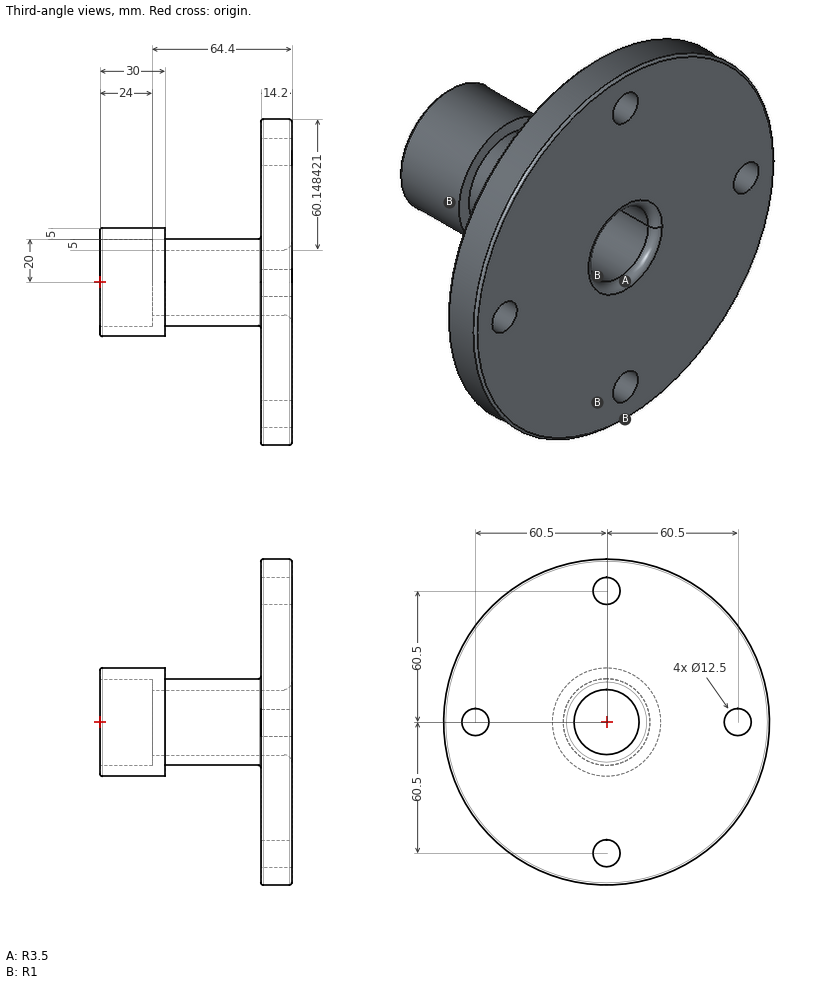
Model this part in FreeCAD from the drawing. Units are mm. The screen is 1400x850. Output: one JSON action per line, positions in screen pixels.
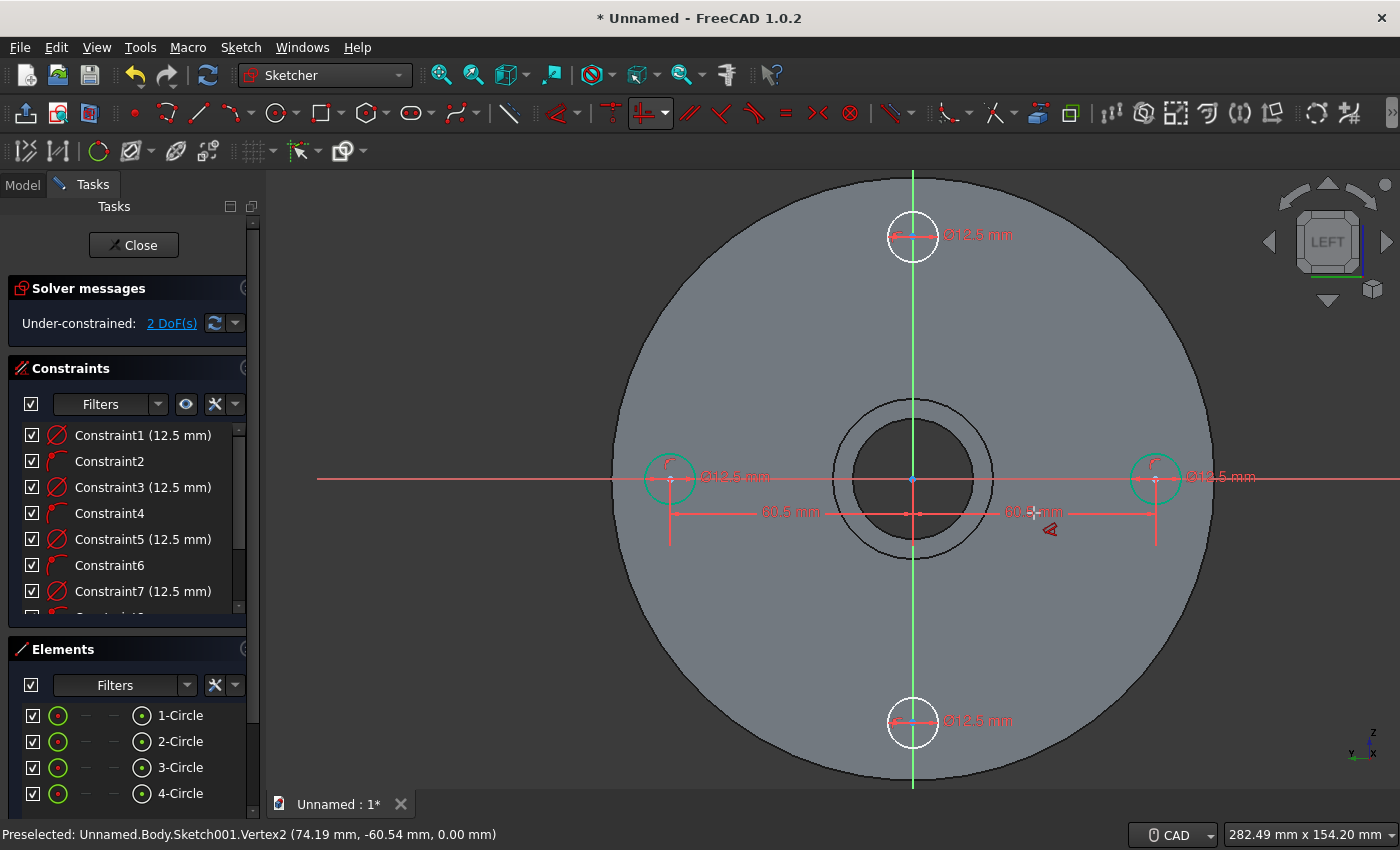
{"action": "left_click", "coordinate": [913, 723]}
{"action": "left_click", "coordinate": [947, 601]}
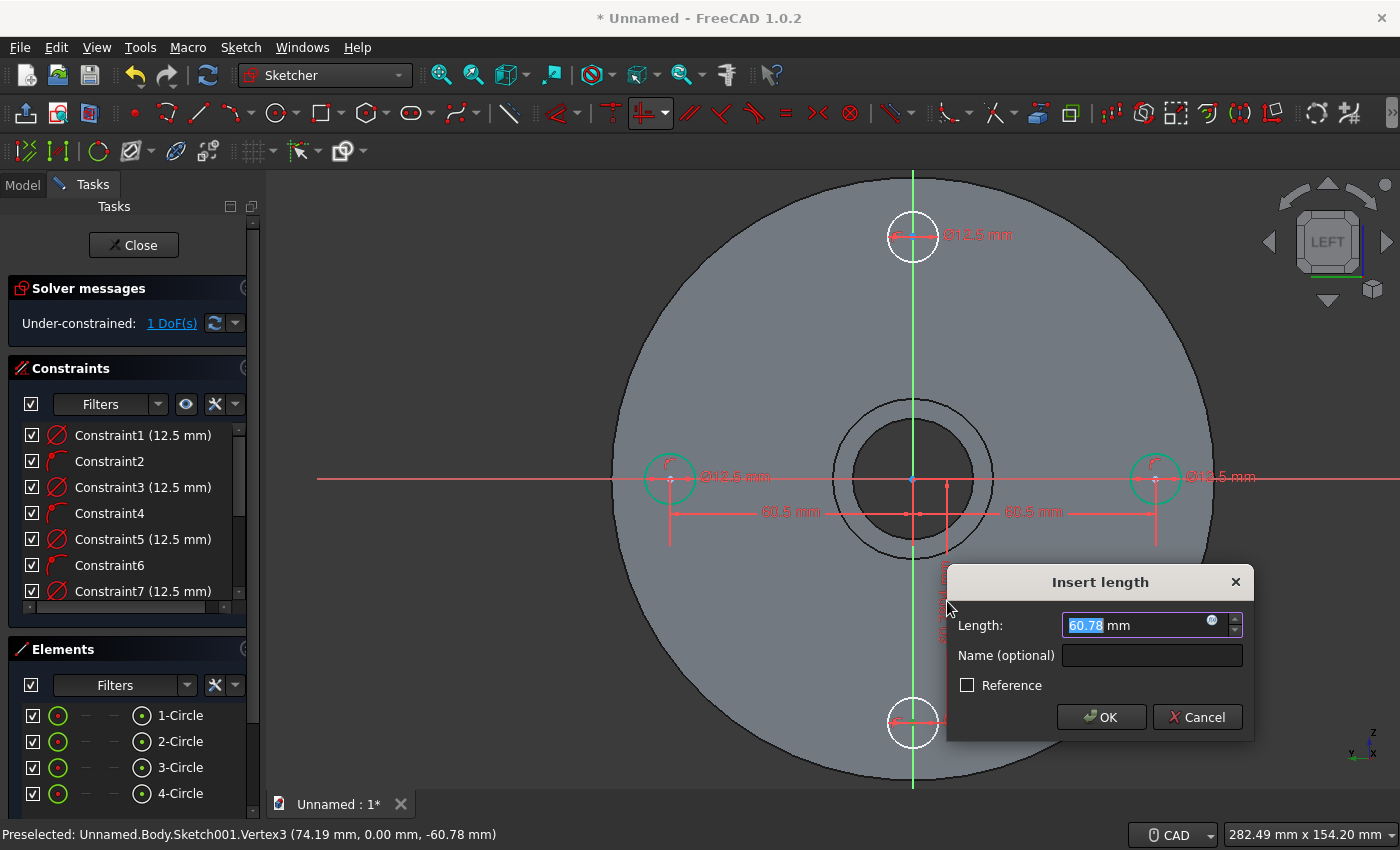
{"action": "type", "text": "60.5"}
{"action": "key", "text": "Return"}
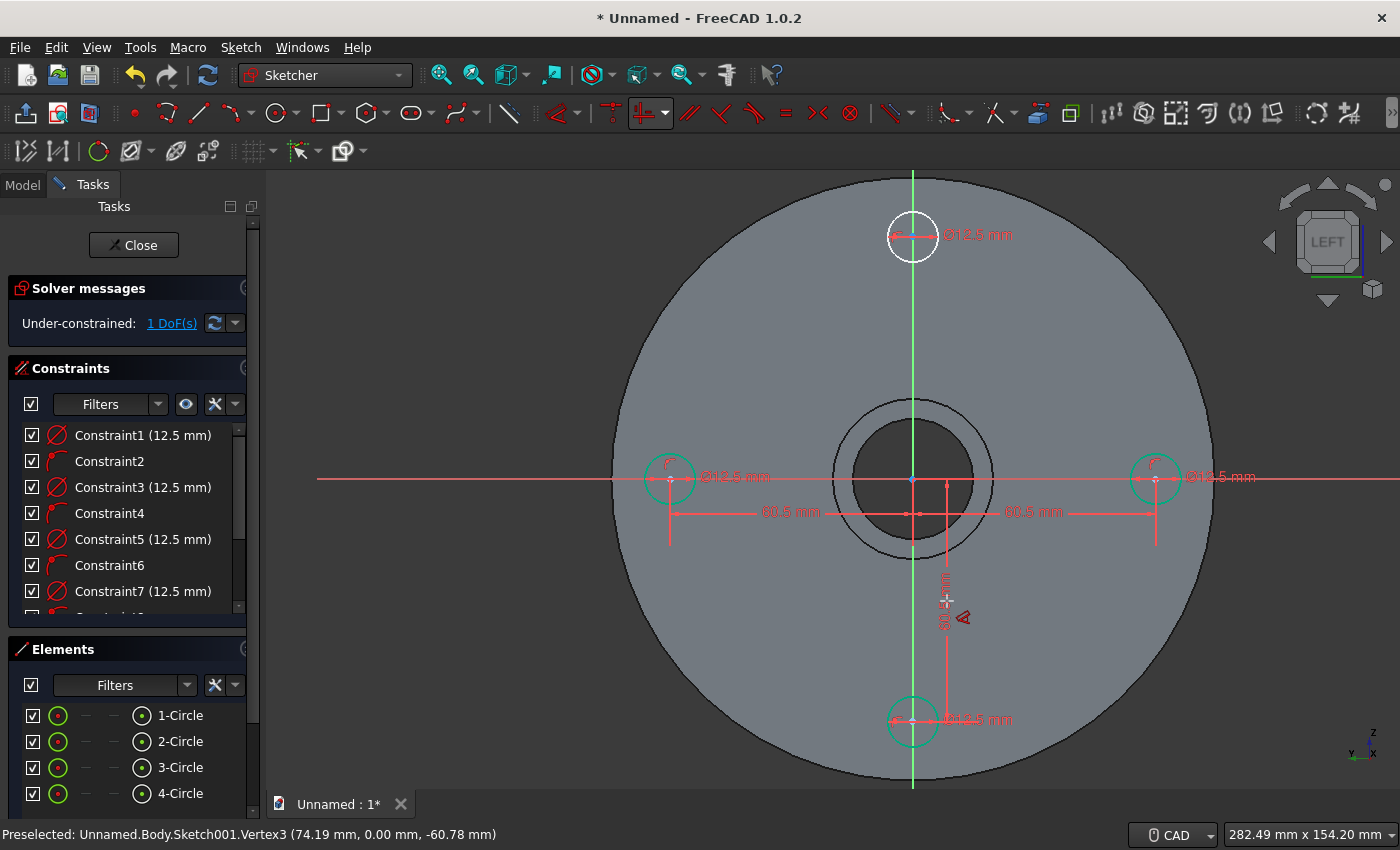
{"action": "left_click", "coordinate": [913, 237]}
{"action": "left_click", "coordinate": [947, 358]}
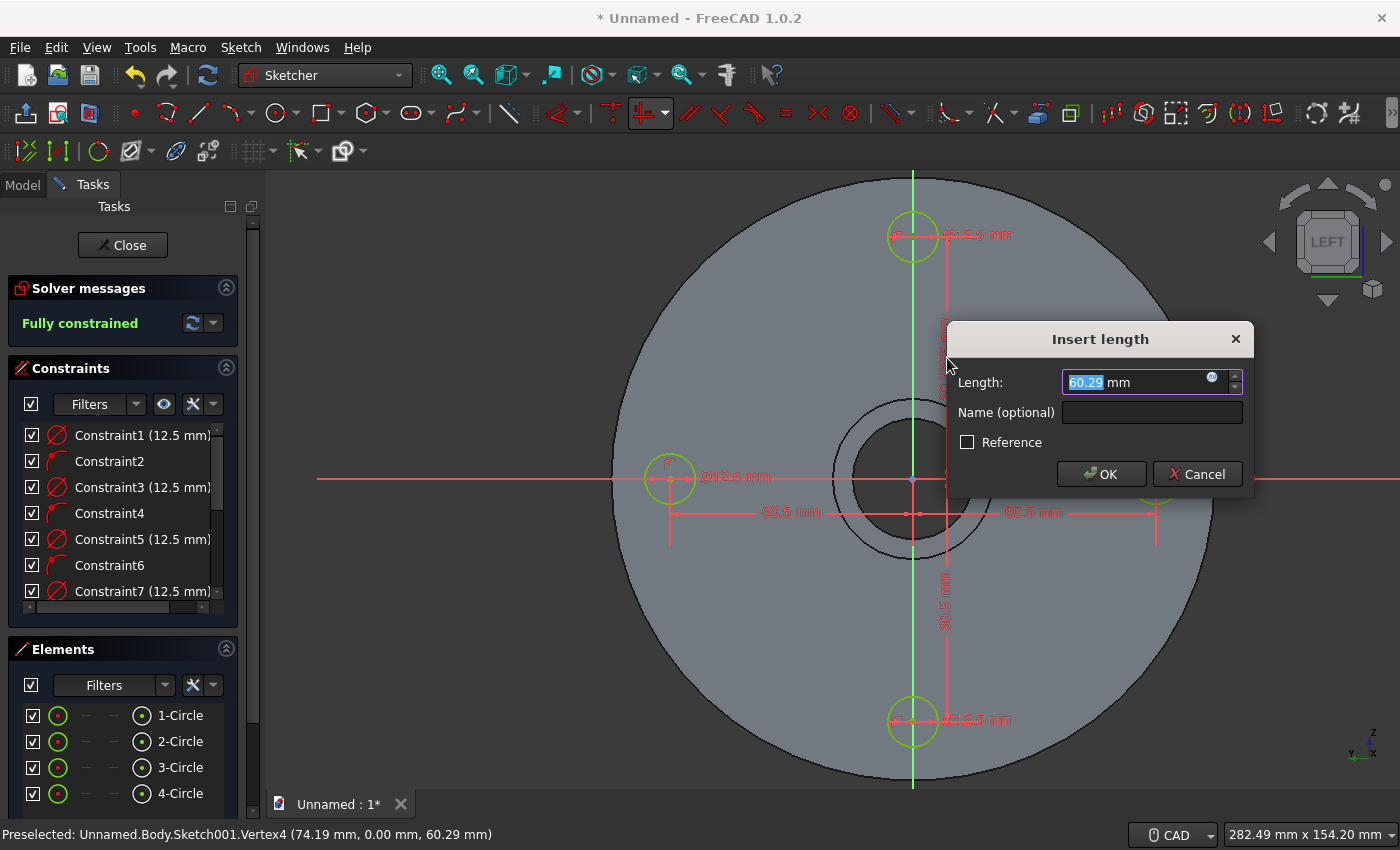
{"action": "type", "text": "60.5"}
{"action": "key", "text": "Return"}
{"action": "key", "text": "Escape"}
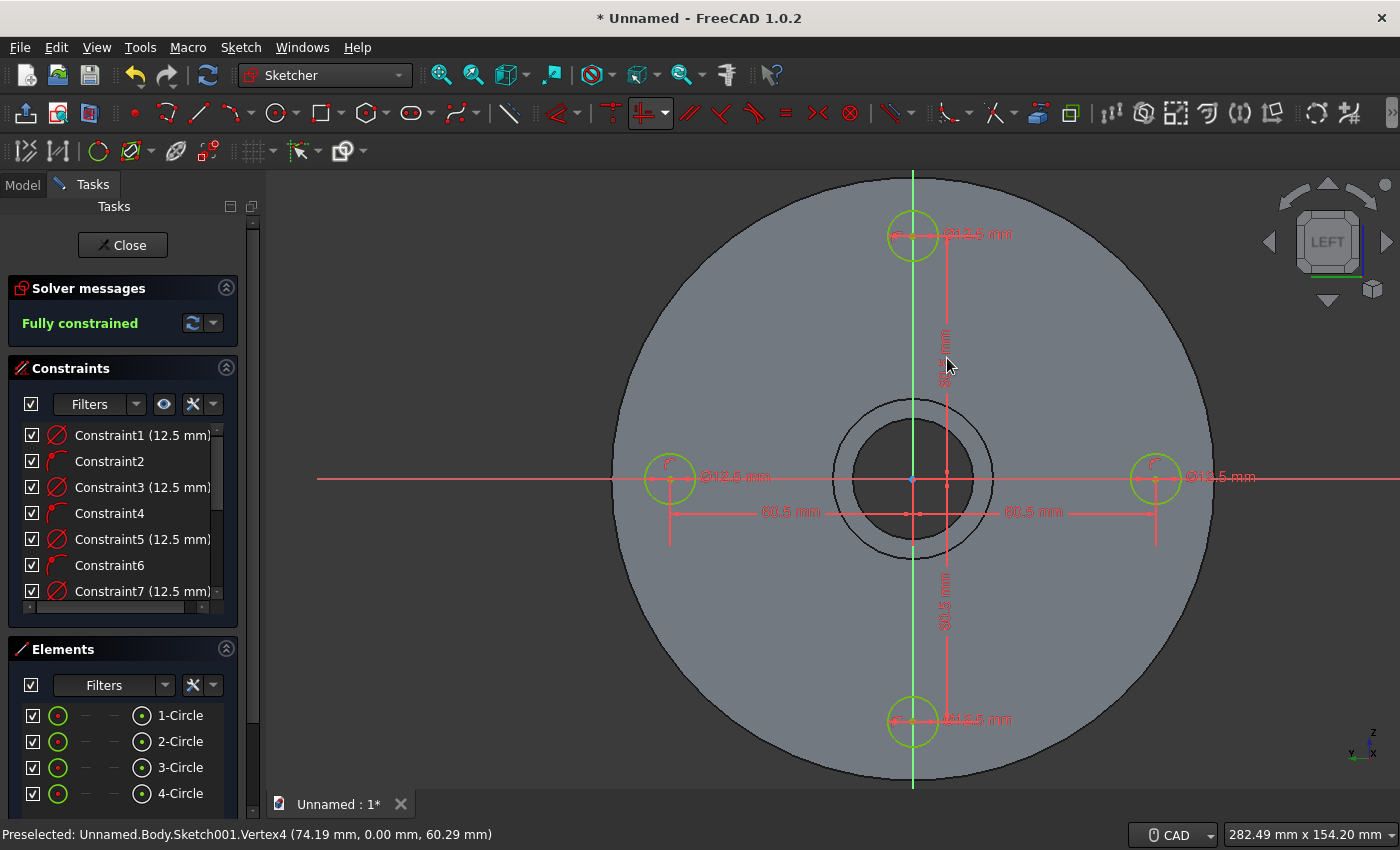
{"action": "left_click", "coordinate": [123, 245]}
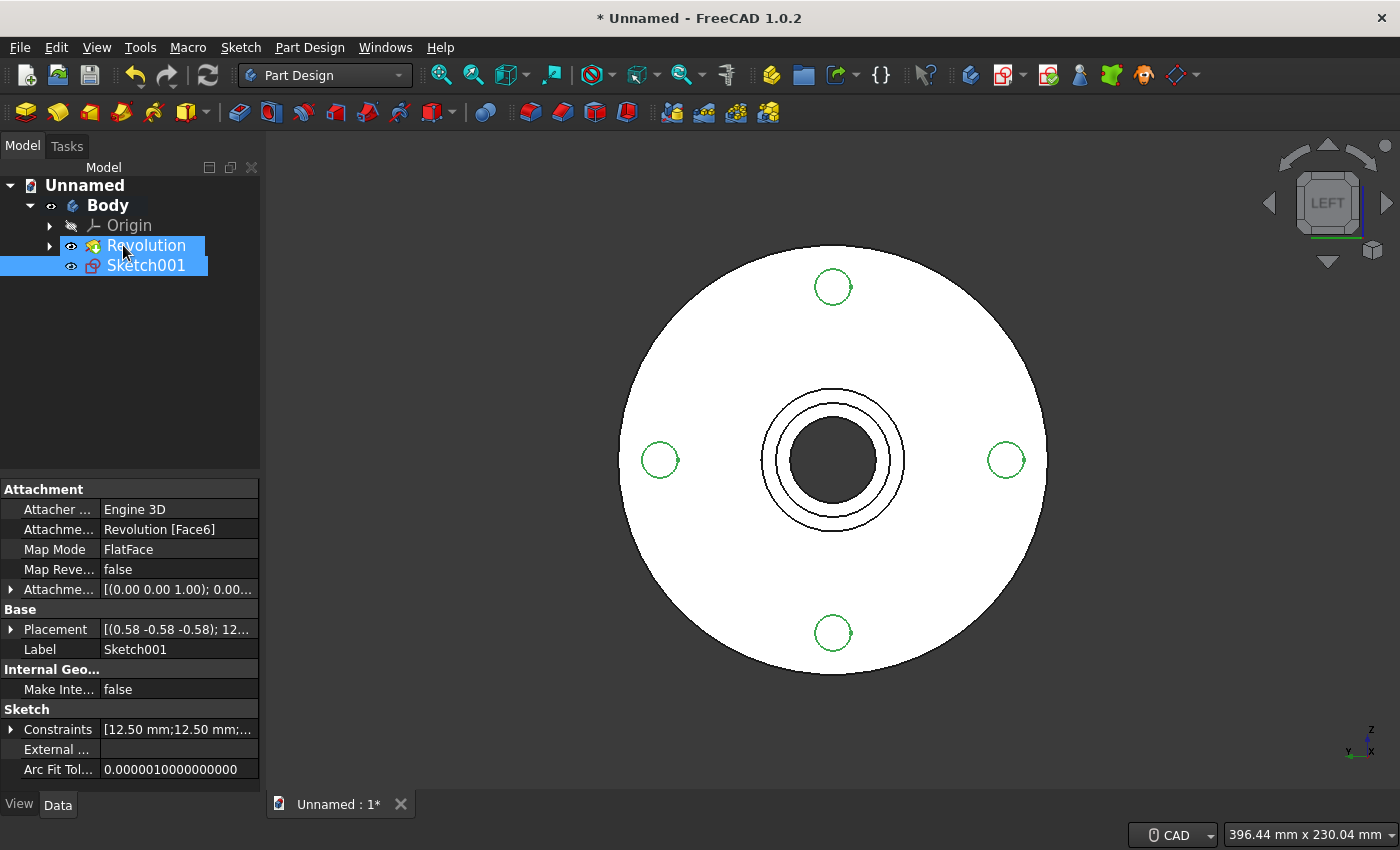
{"action": "left_click", "coordinate": [240, 112]}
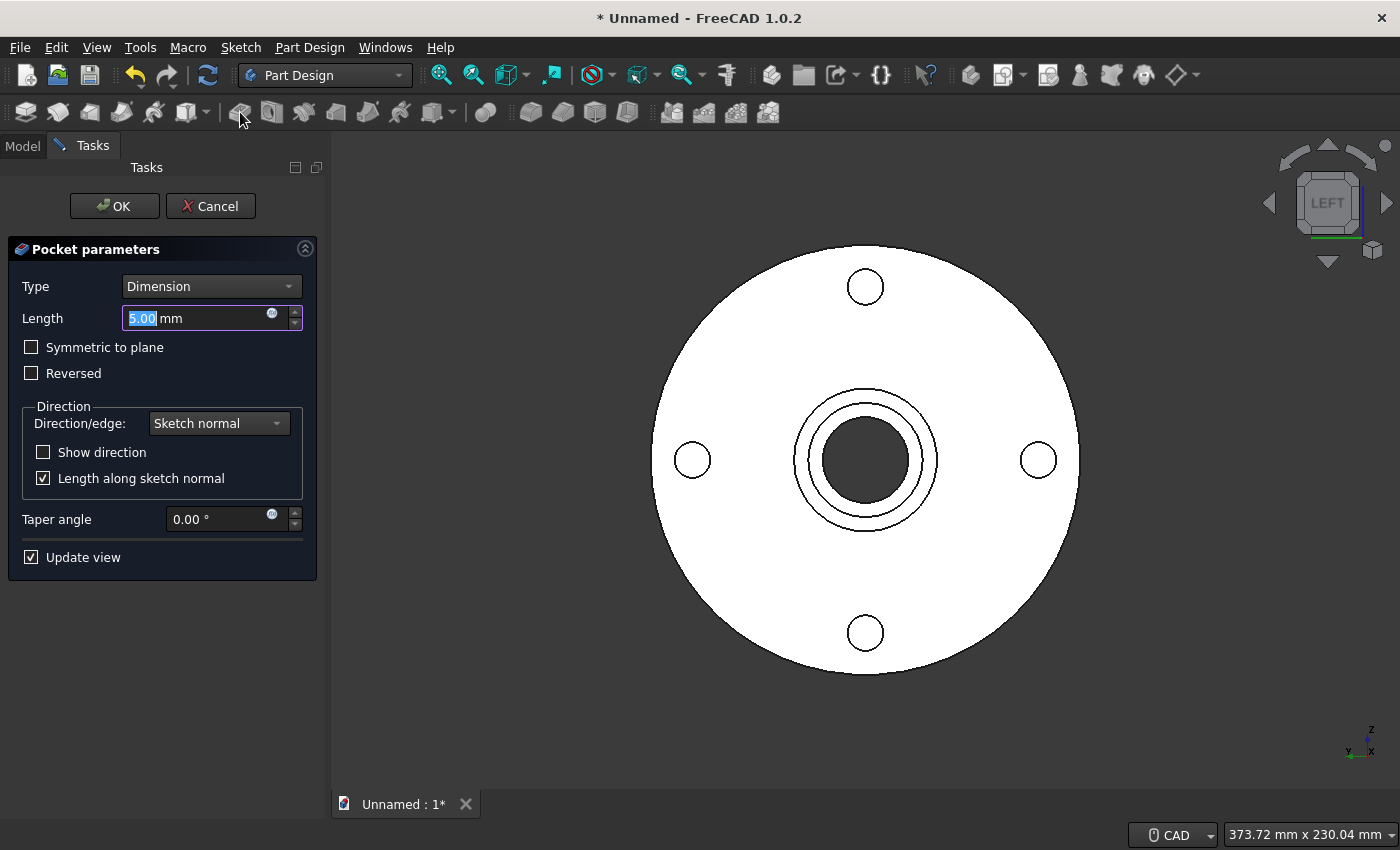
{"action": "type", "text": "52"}
{"action": "key", "text": "Tab"}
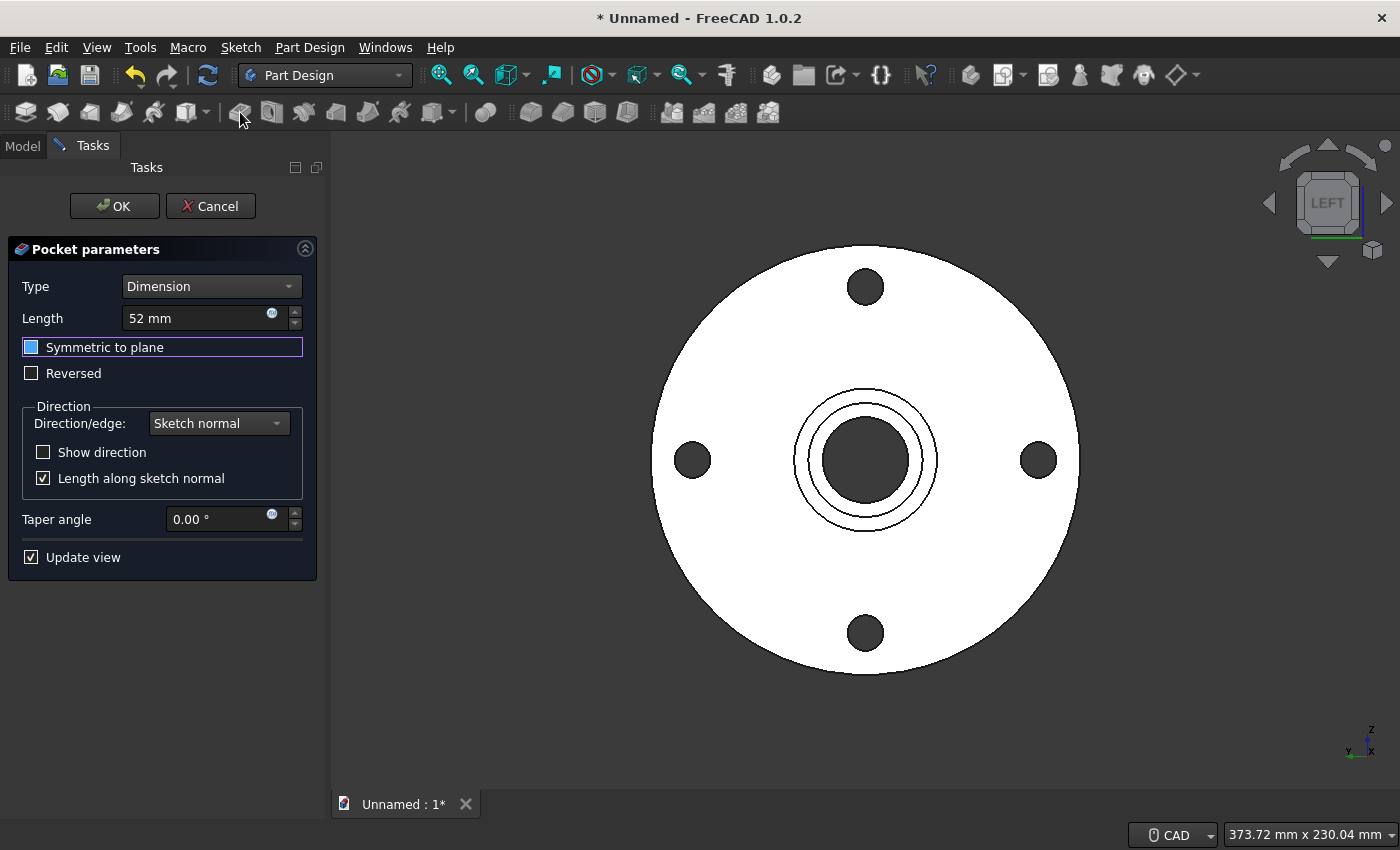
{"action": "left_click", "coordinate": [115, 206]}